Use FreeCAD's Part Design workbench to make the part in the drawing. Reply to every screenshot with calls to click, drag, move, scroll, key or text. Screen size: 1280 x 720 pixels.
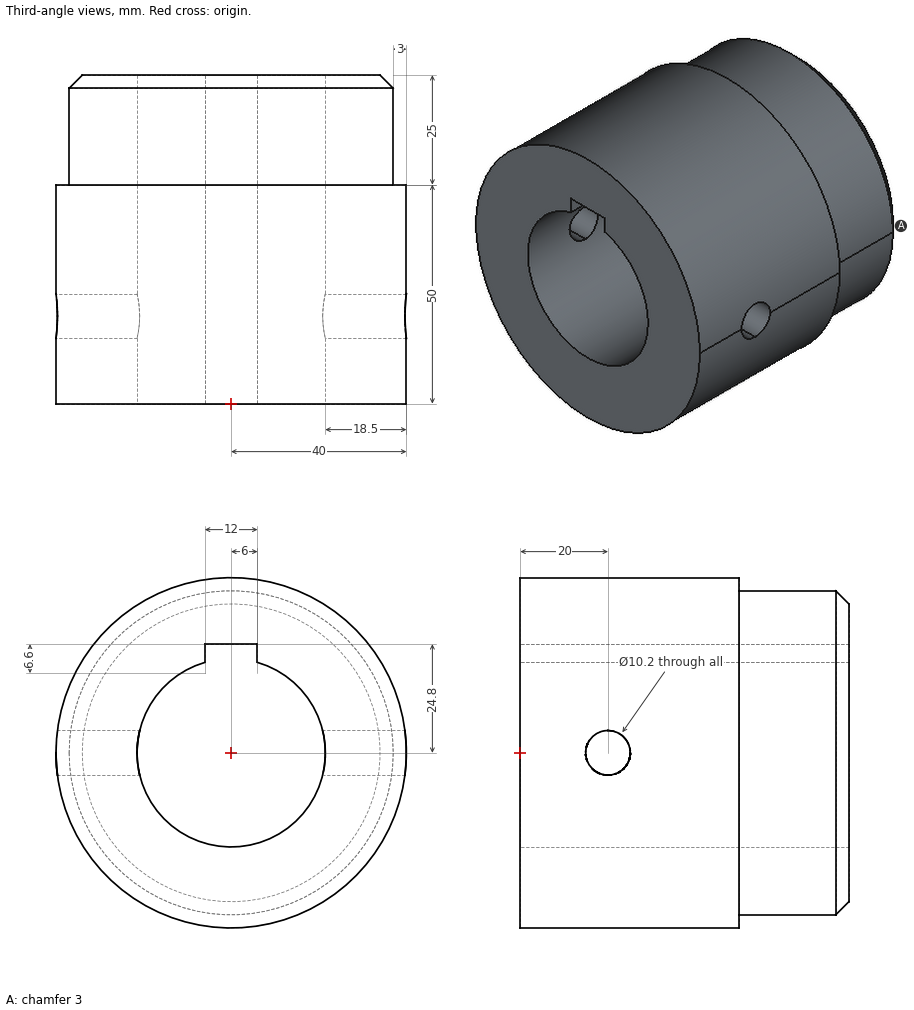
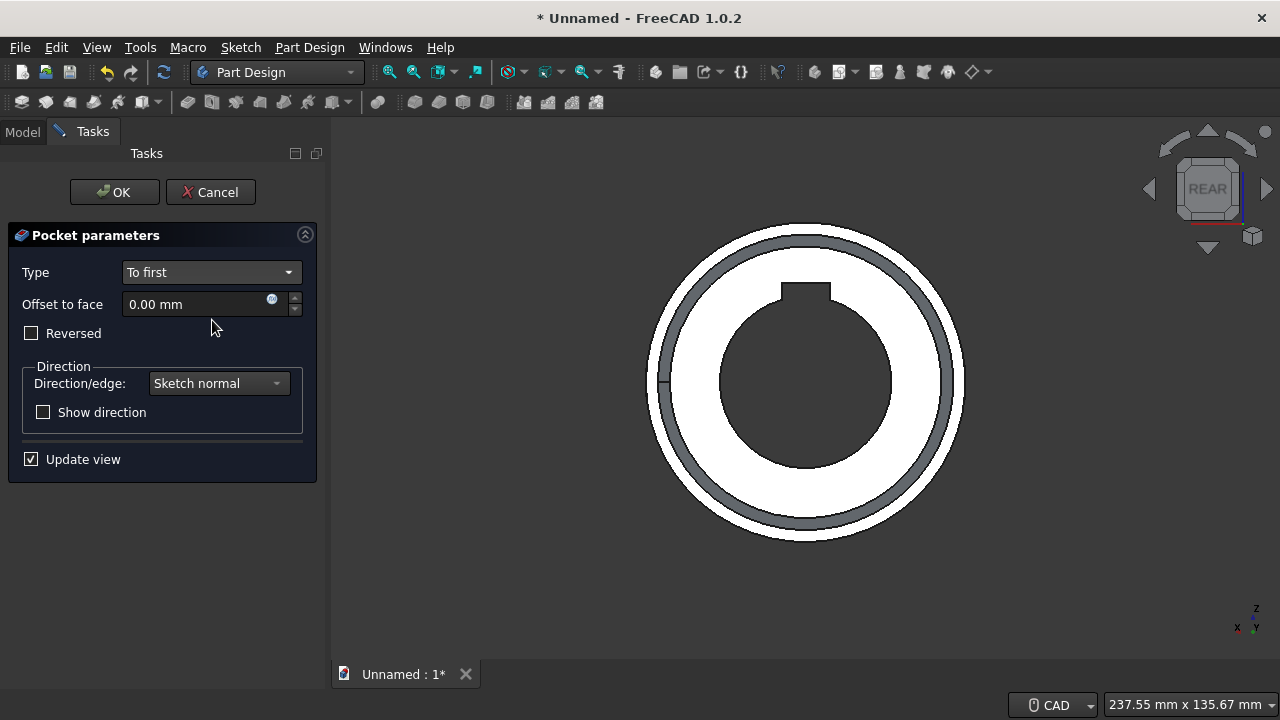
click(115, 192)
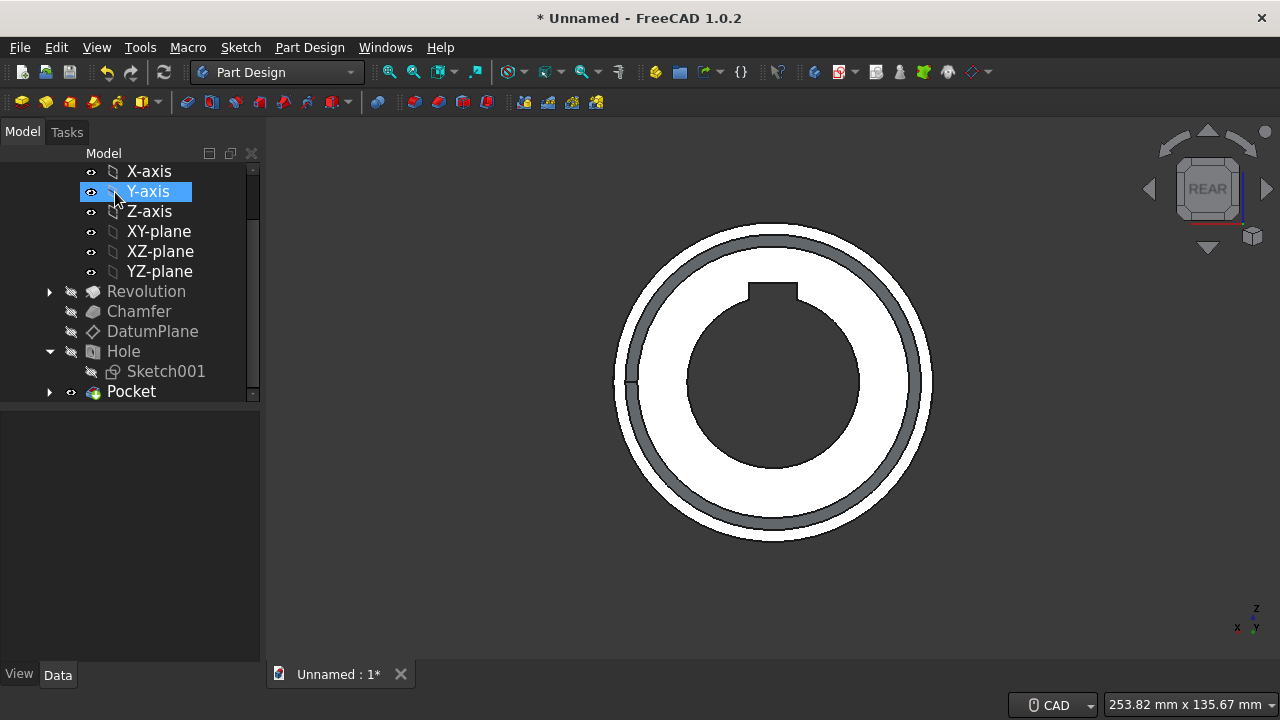
key(0)